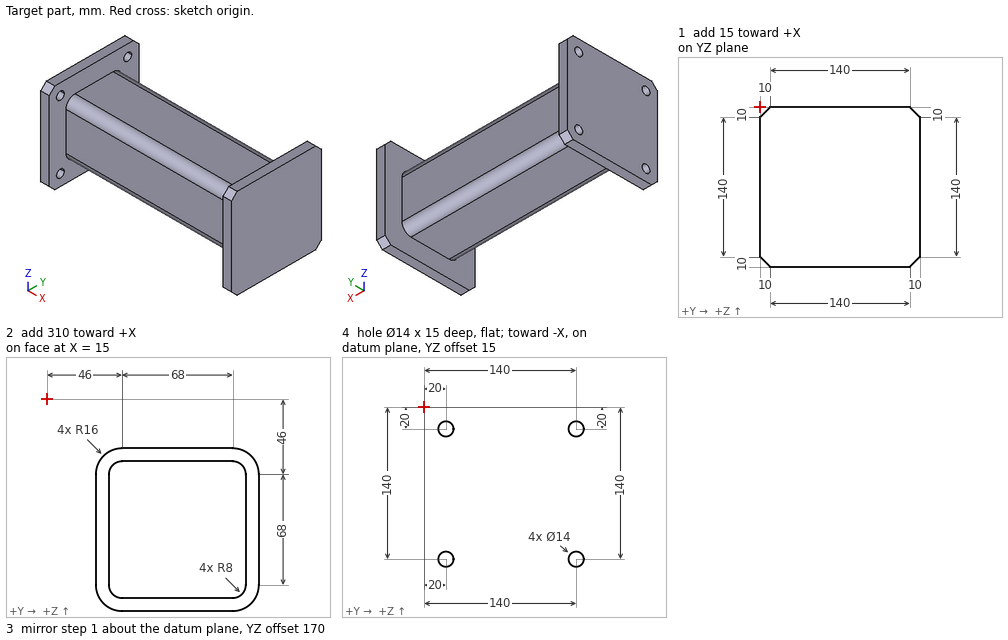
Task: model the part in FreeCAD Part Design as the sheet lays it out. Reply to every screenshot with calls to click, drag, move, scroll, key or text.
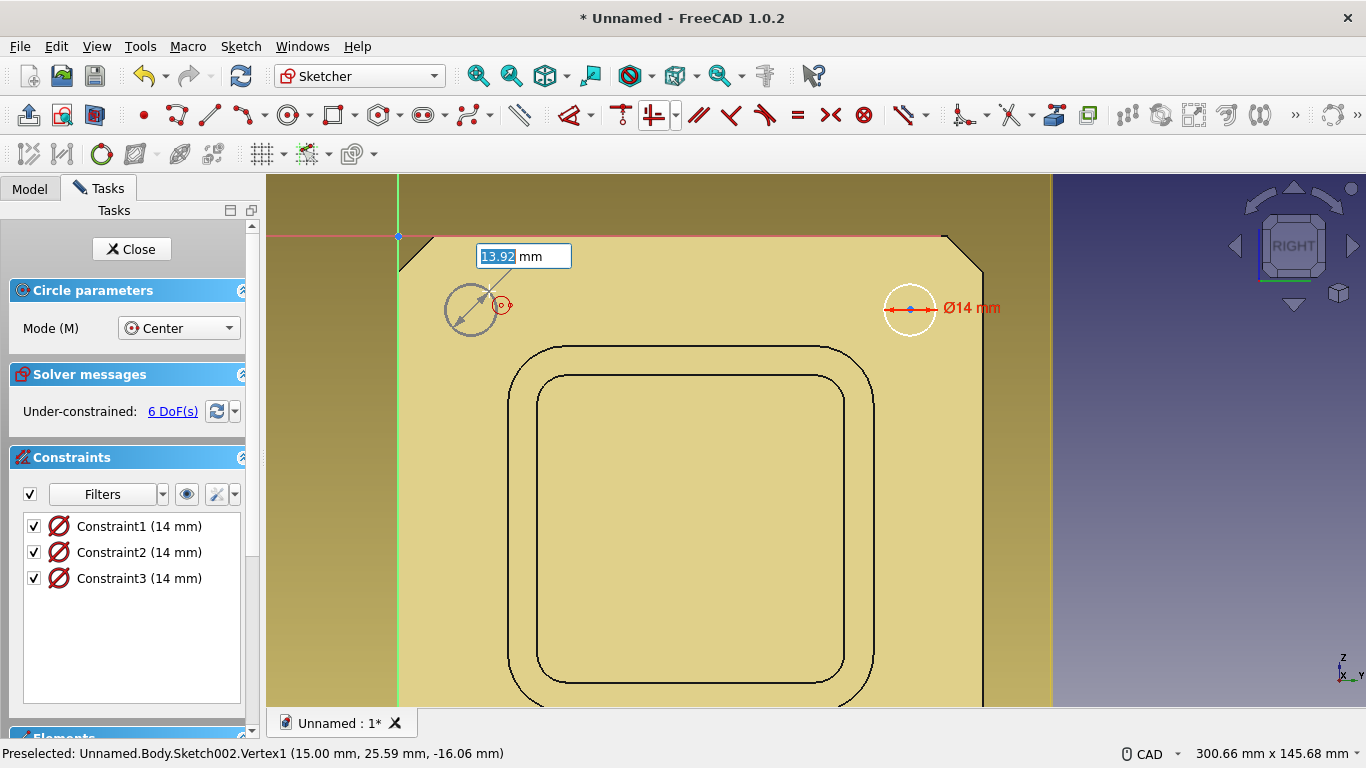
text(14)
key(Return)
key(Escape)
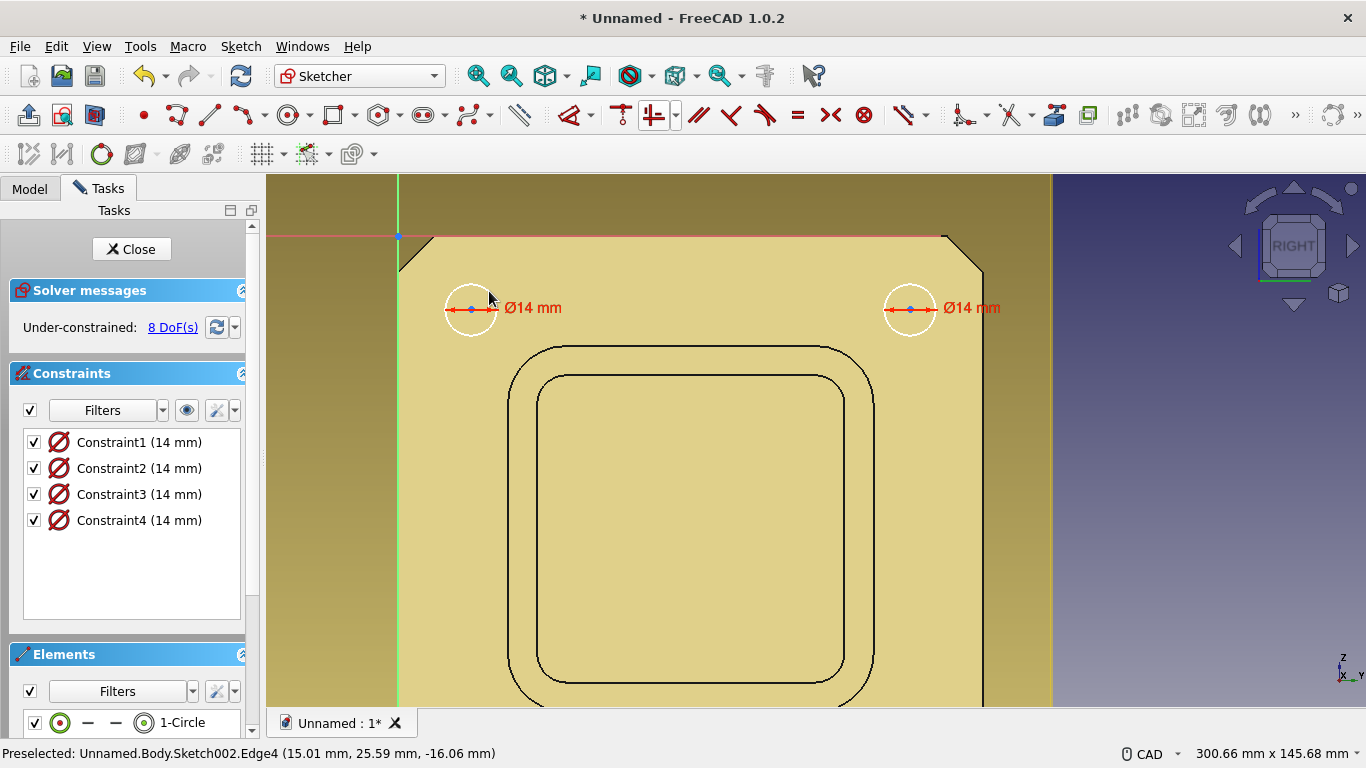
click(568, 116)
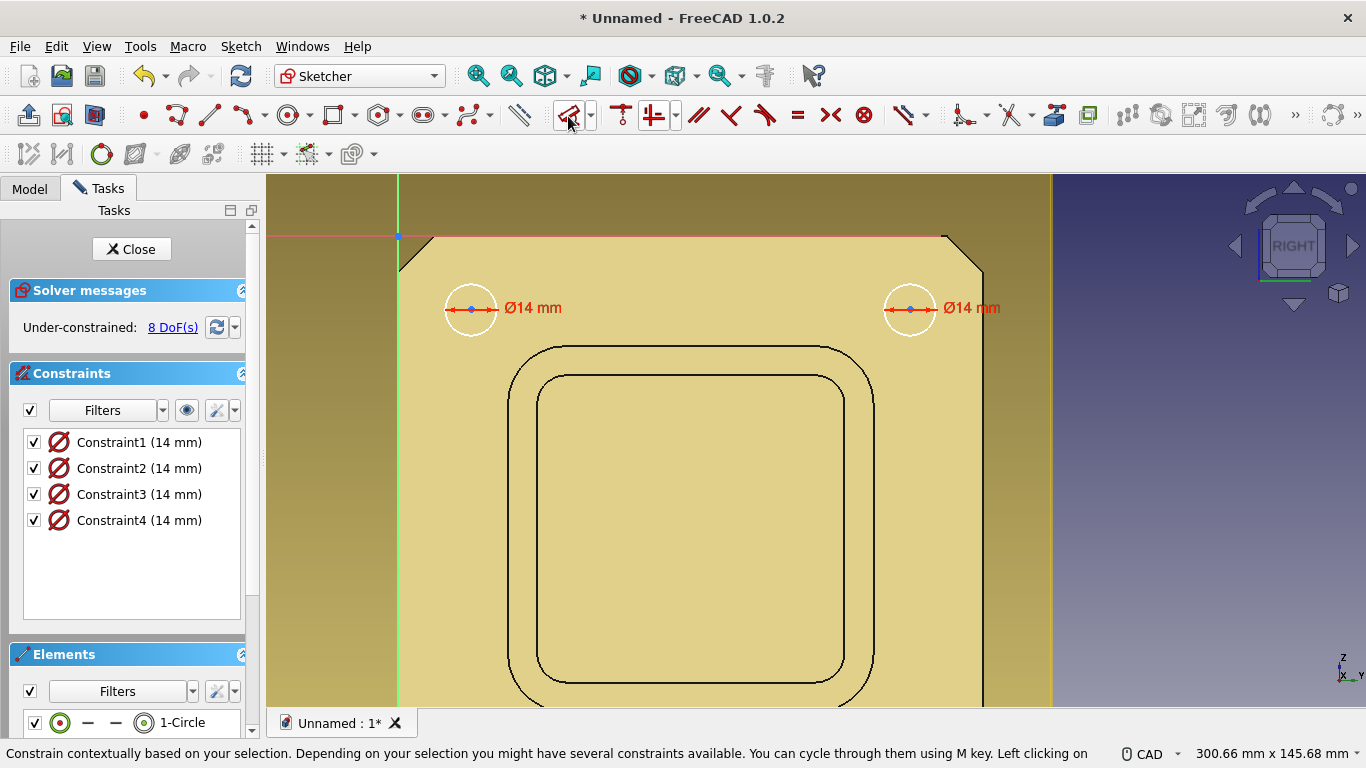
scroll(911, 309, down, 2)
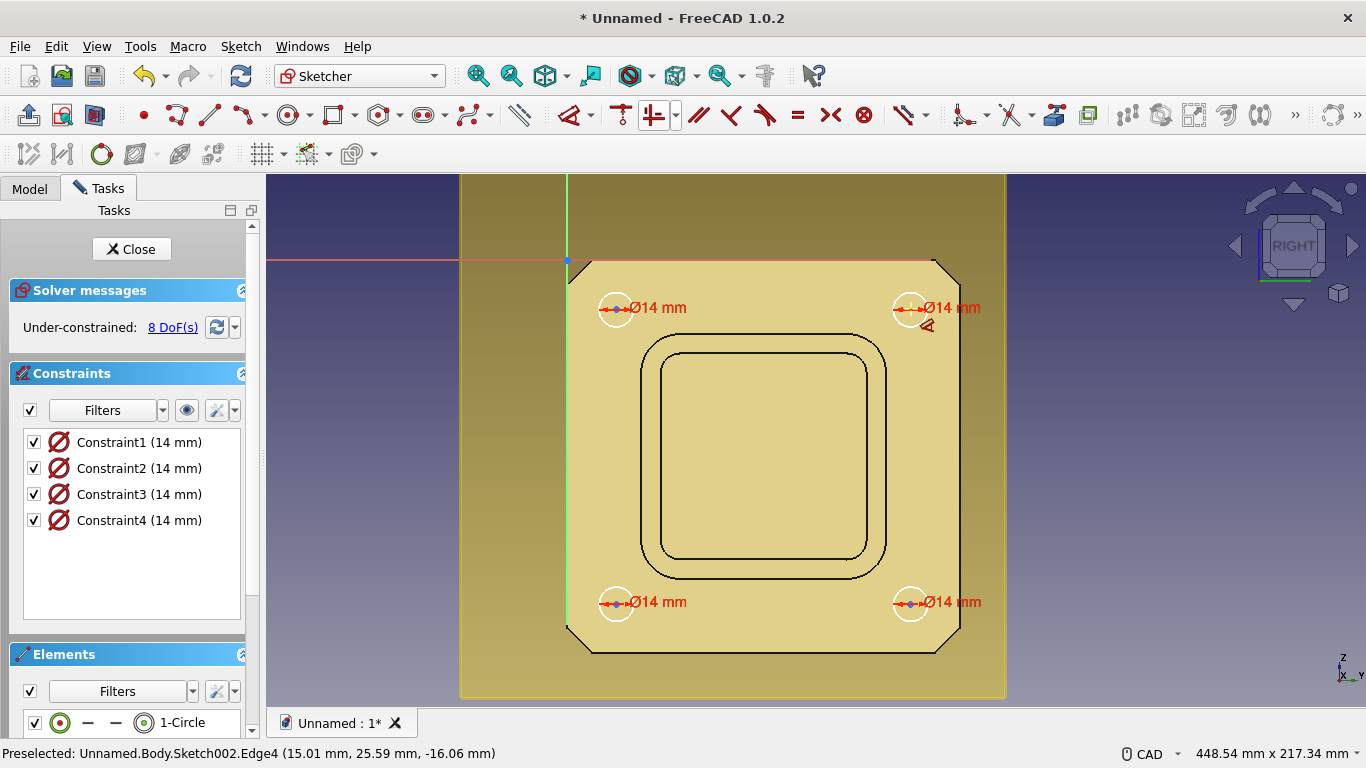
click(617, 604)
click(592, 226)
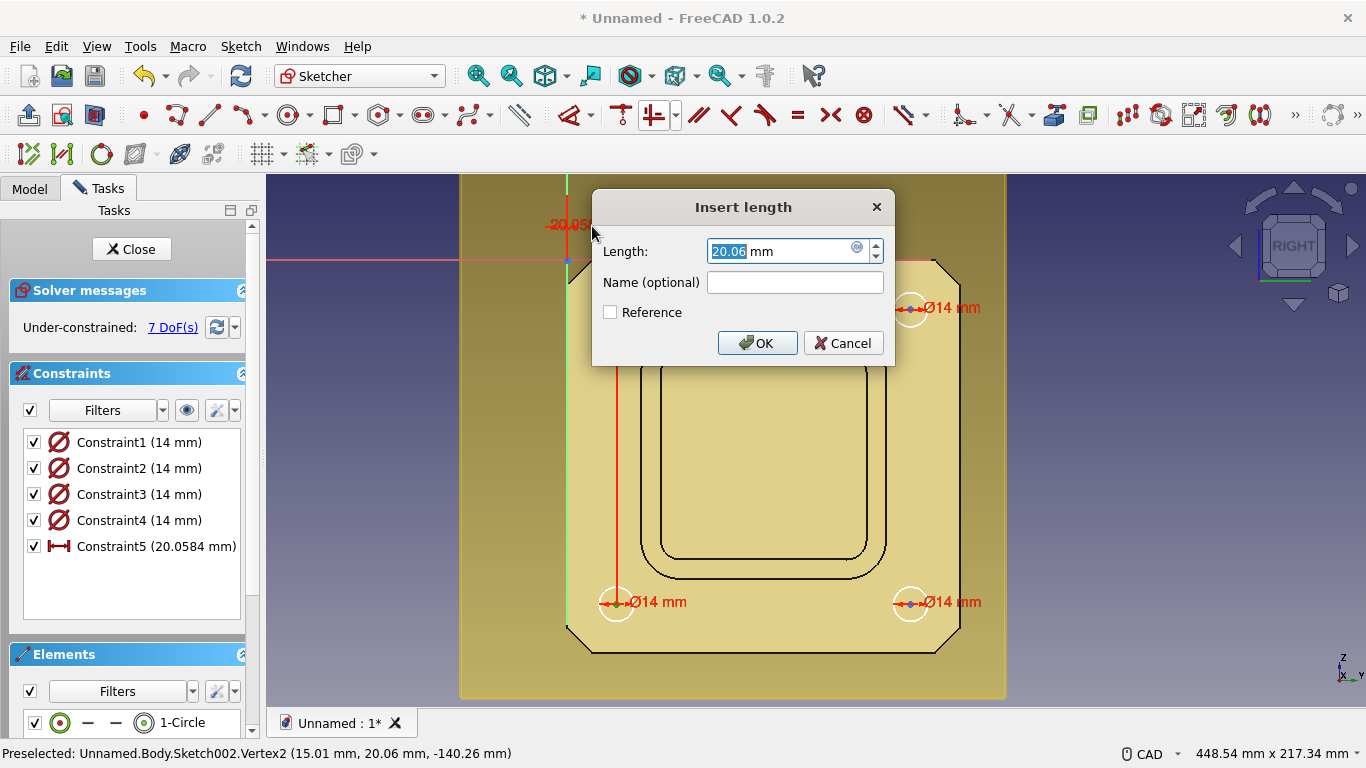
text(20)
key(Return)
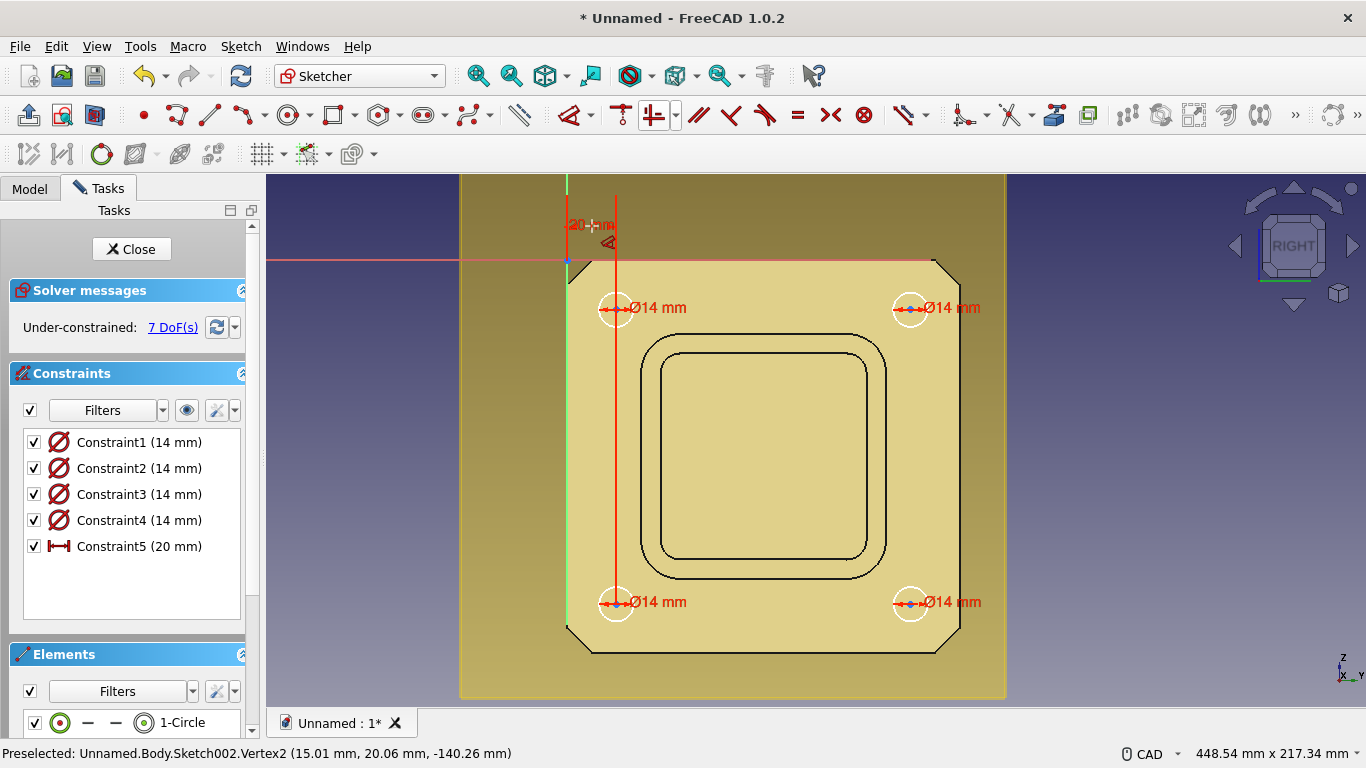
click(911, 310)
click(533, 285)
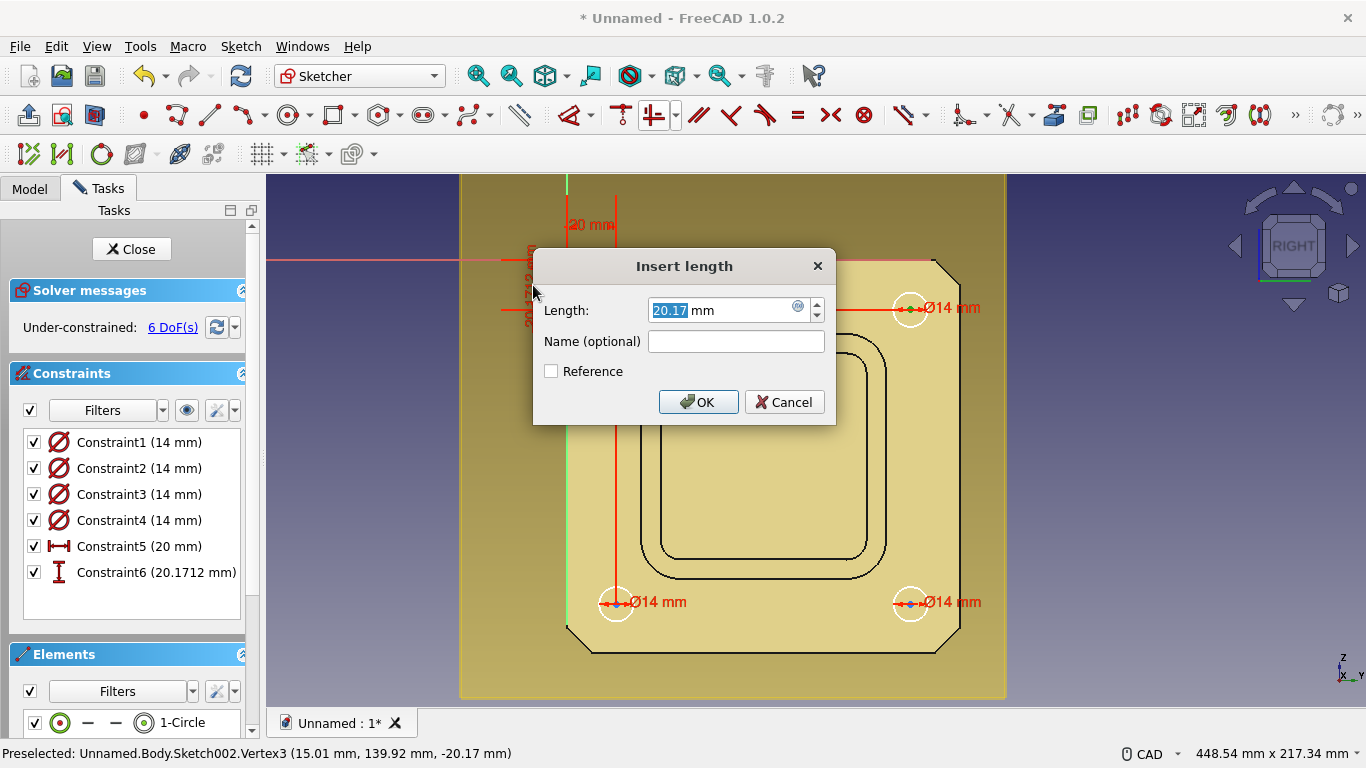
text(20)
key(Return)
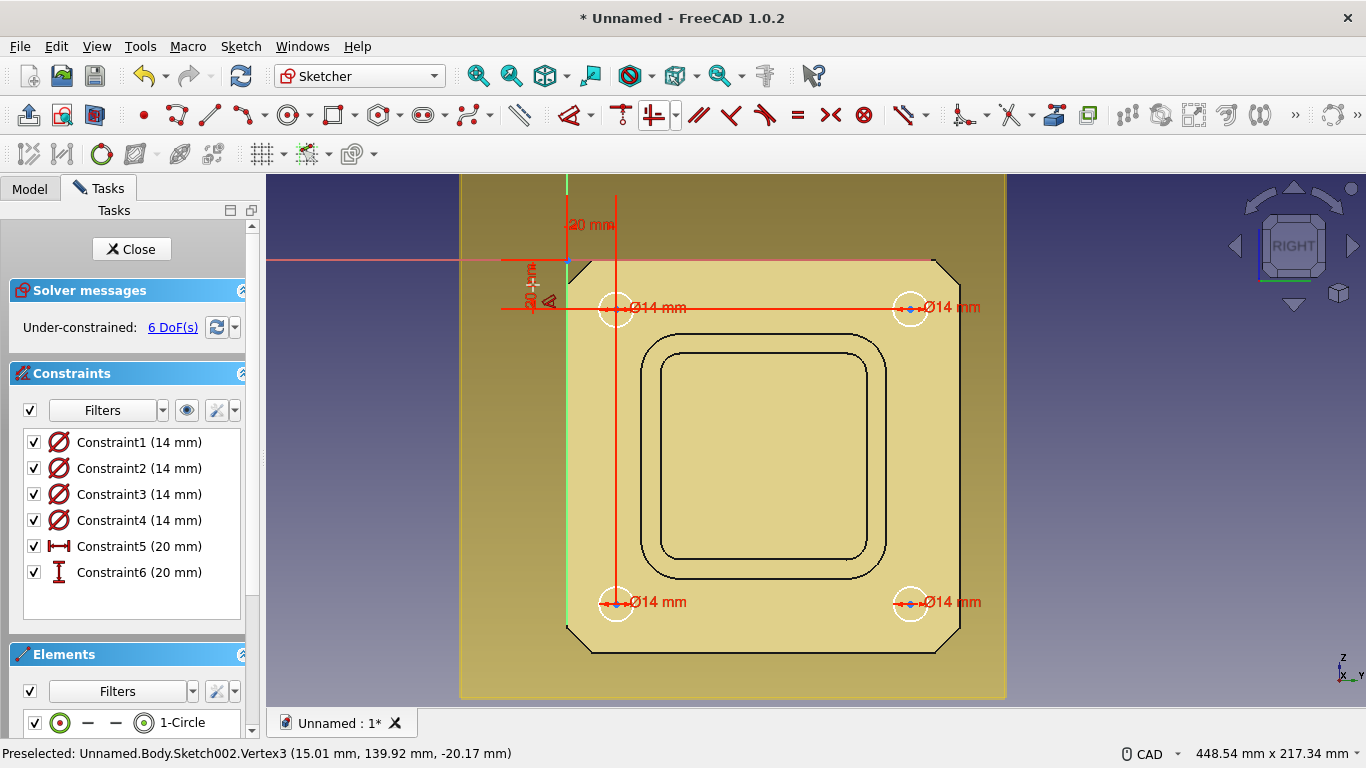
click(616, 310)
click(592, 344)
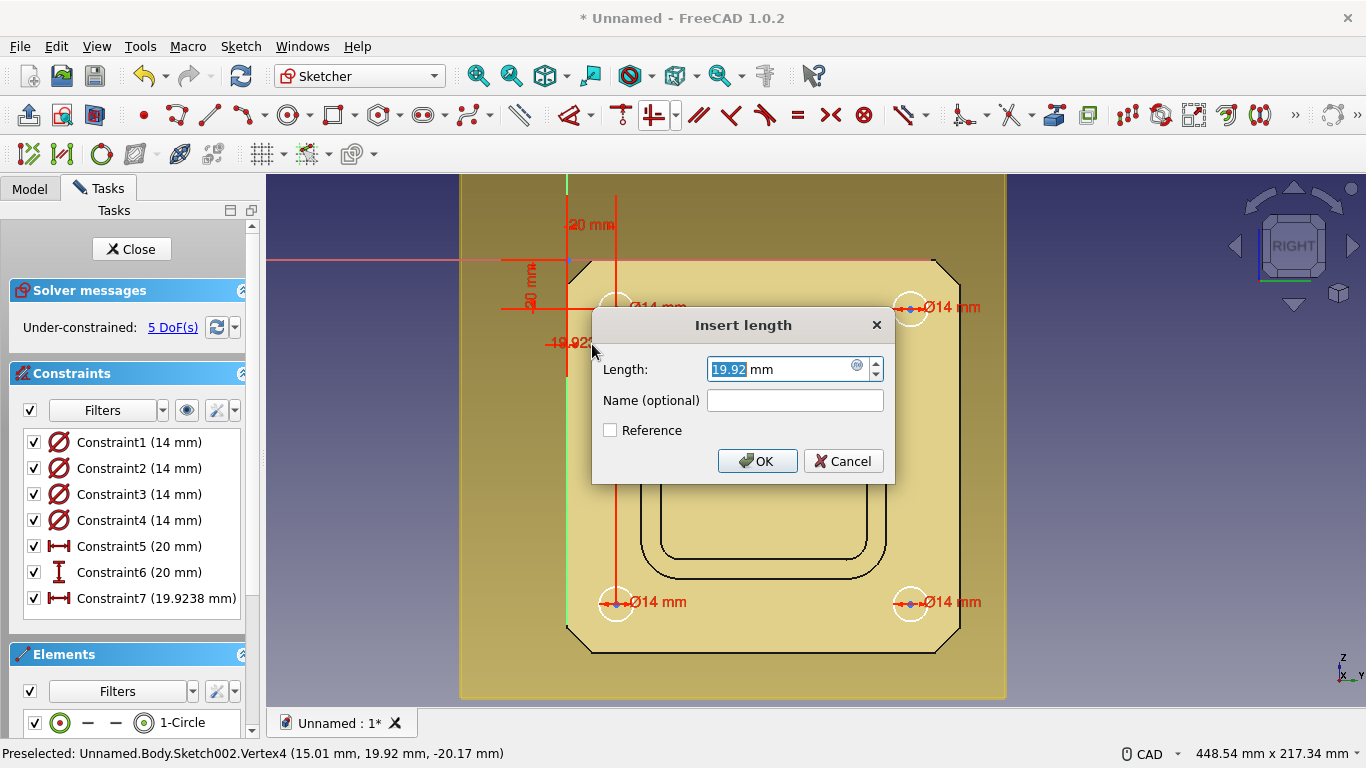
text(20)
key(Return)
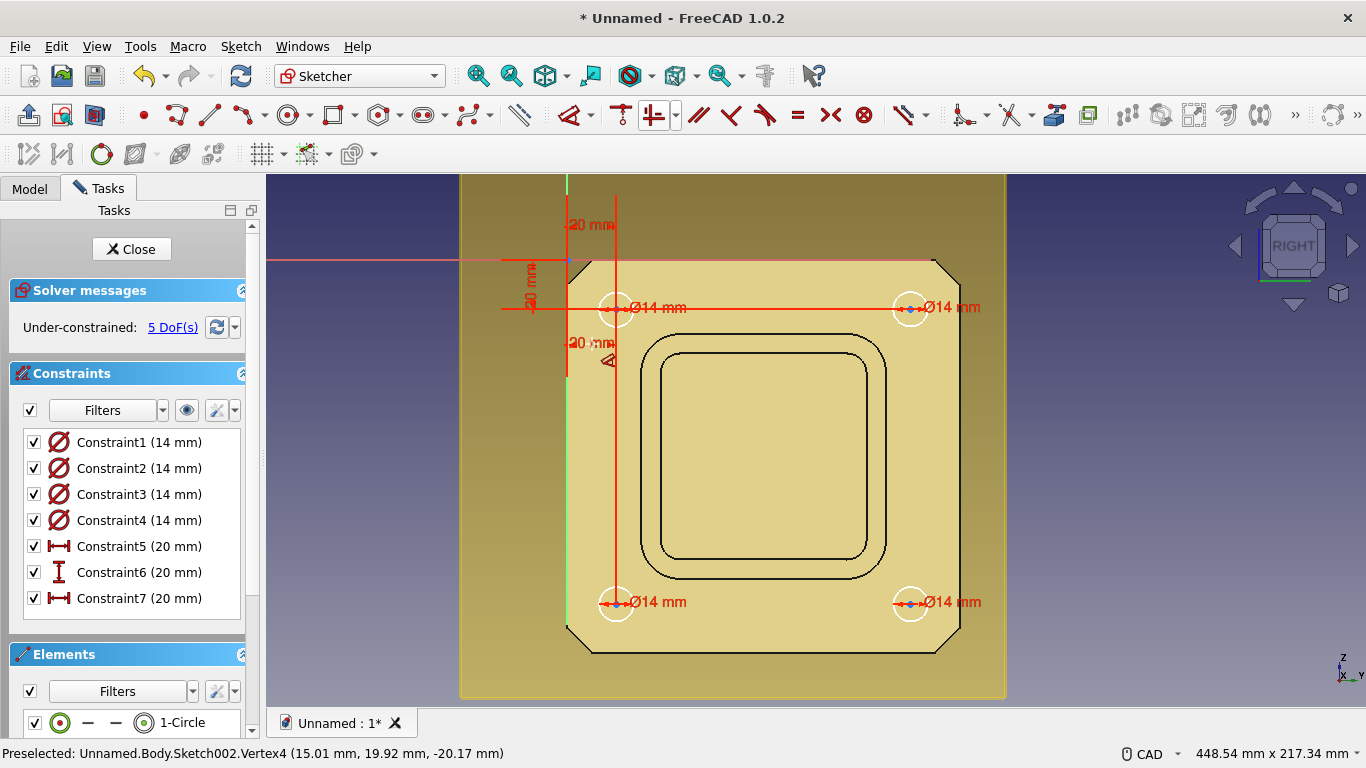
click(616, 310)
click(650, 285)